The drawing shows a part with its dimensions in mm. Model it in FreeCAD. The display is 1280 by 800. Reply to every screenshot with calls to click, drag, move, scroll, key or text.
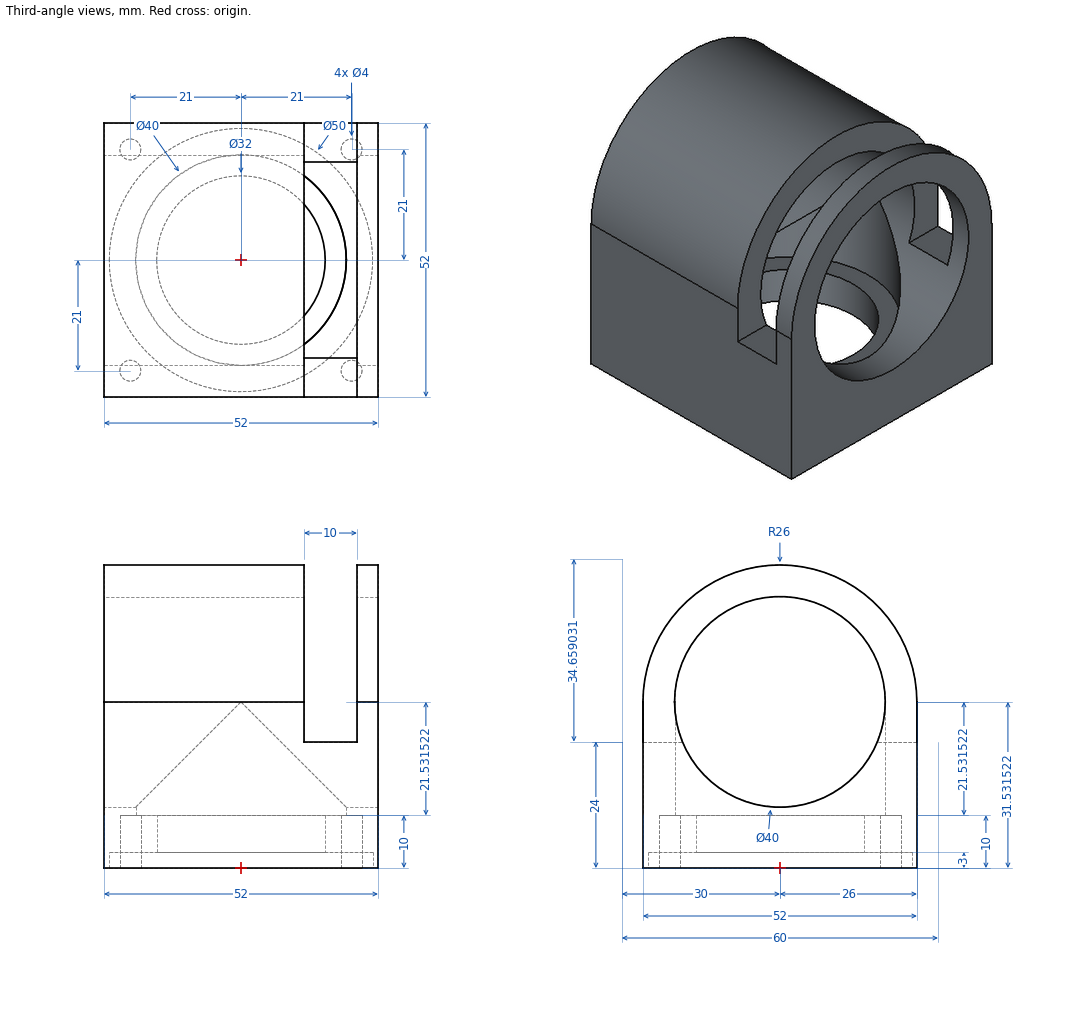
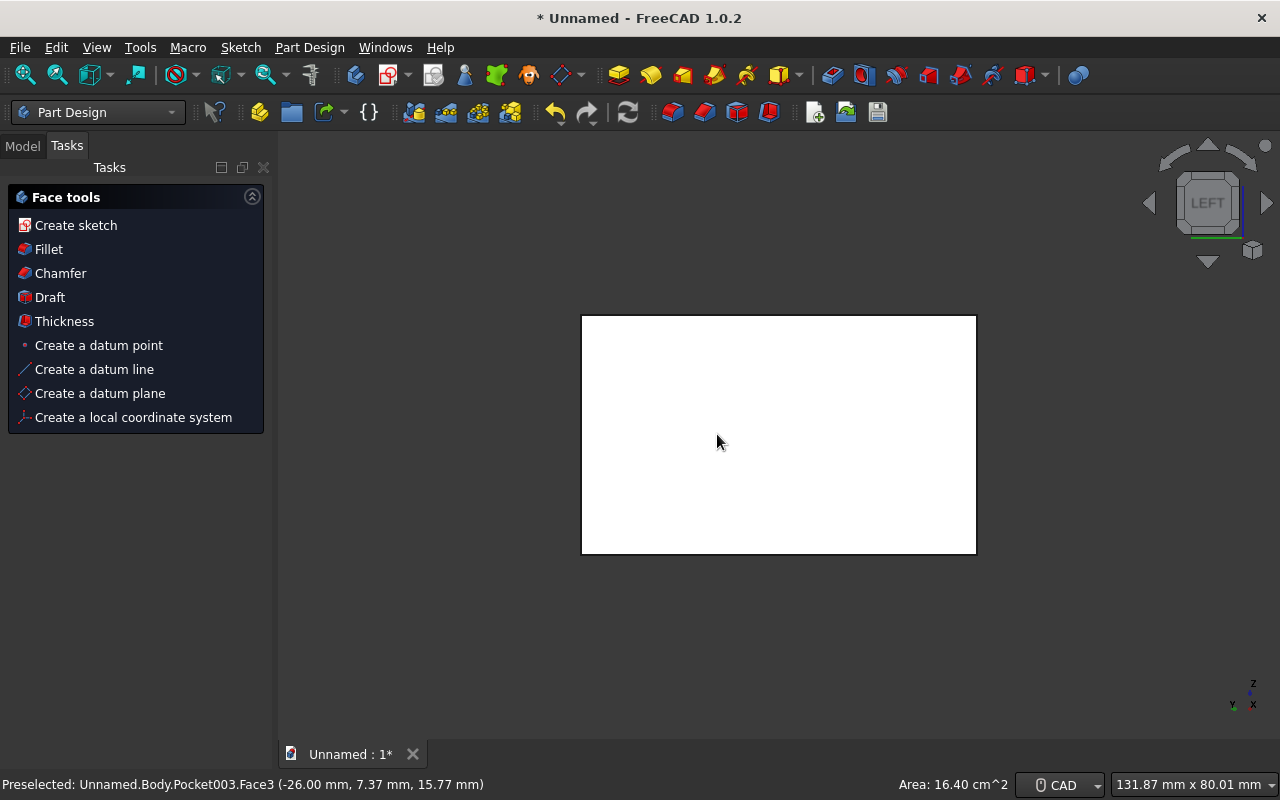
click(388, 76)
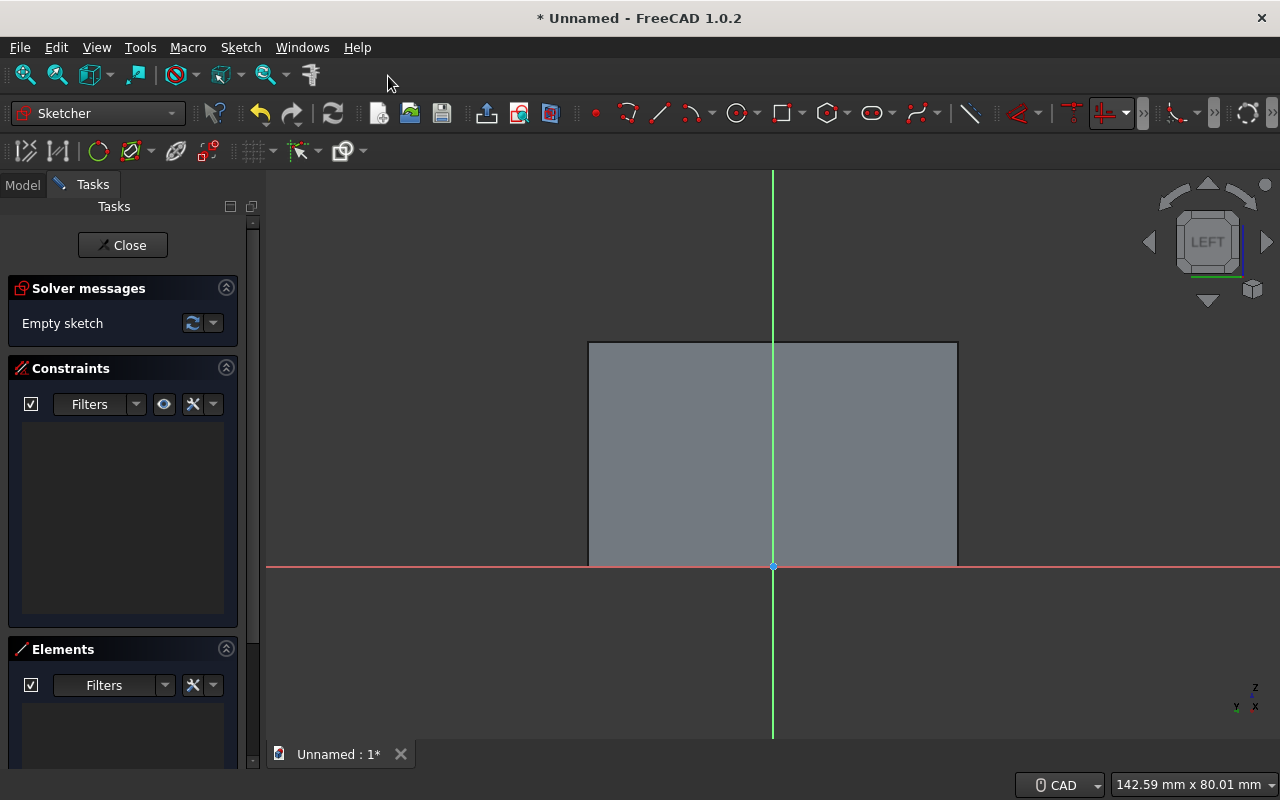
scroll(395, 711, down, 1)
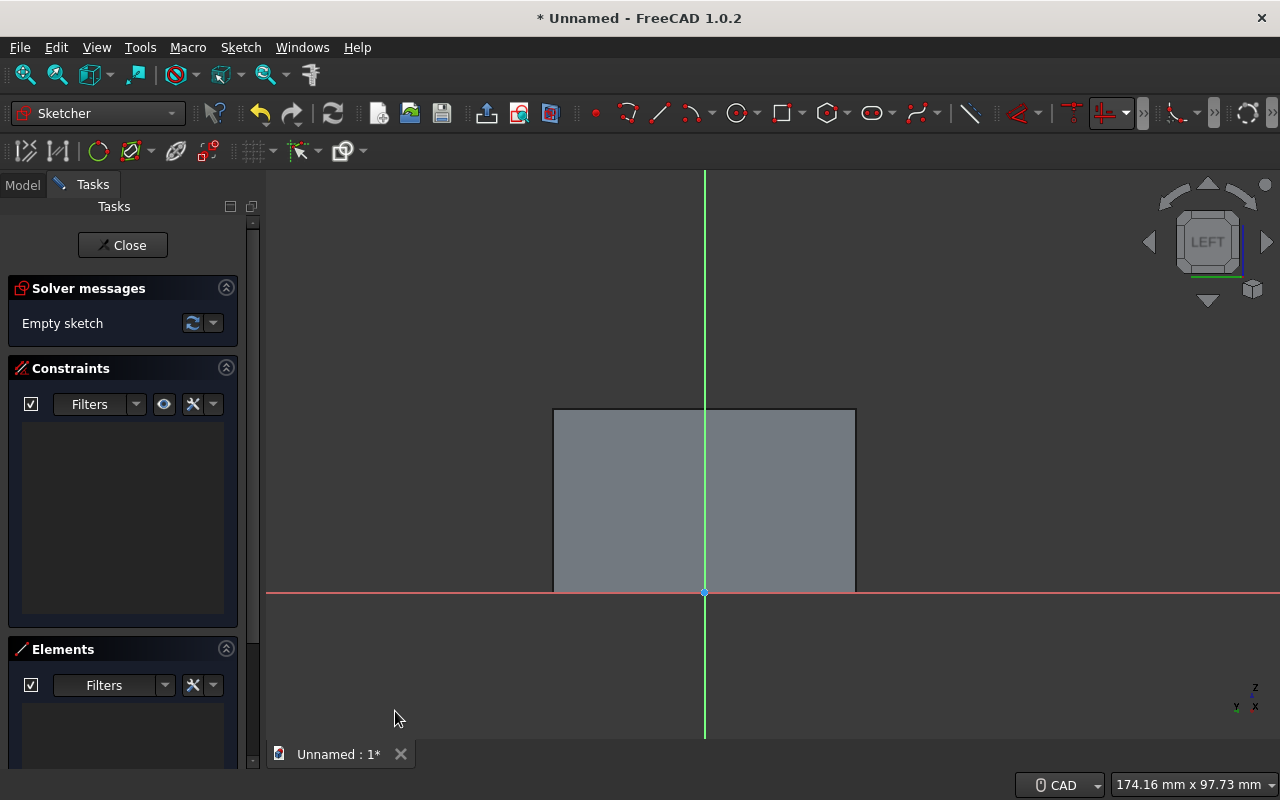
click(660, 114)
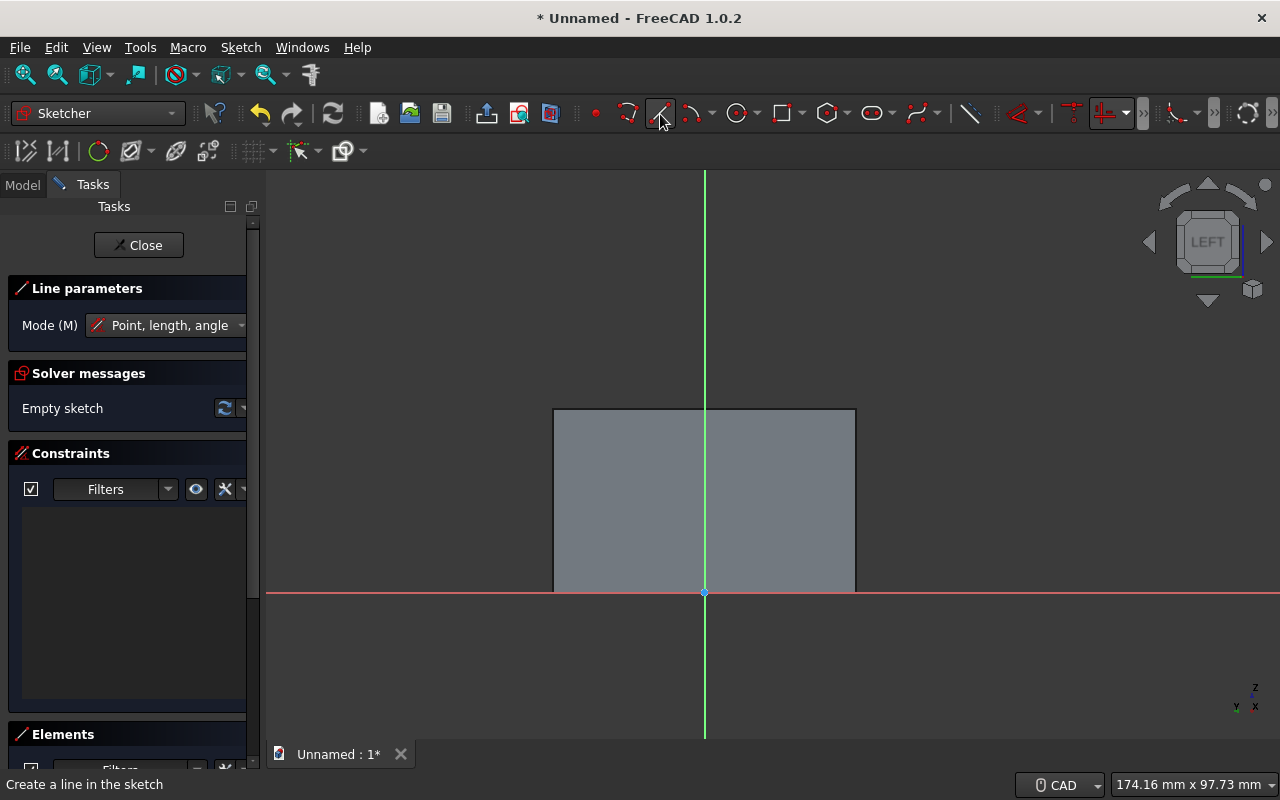
click(553, 409)
click(856, 409)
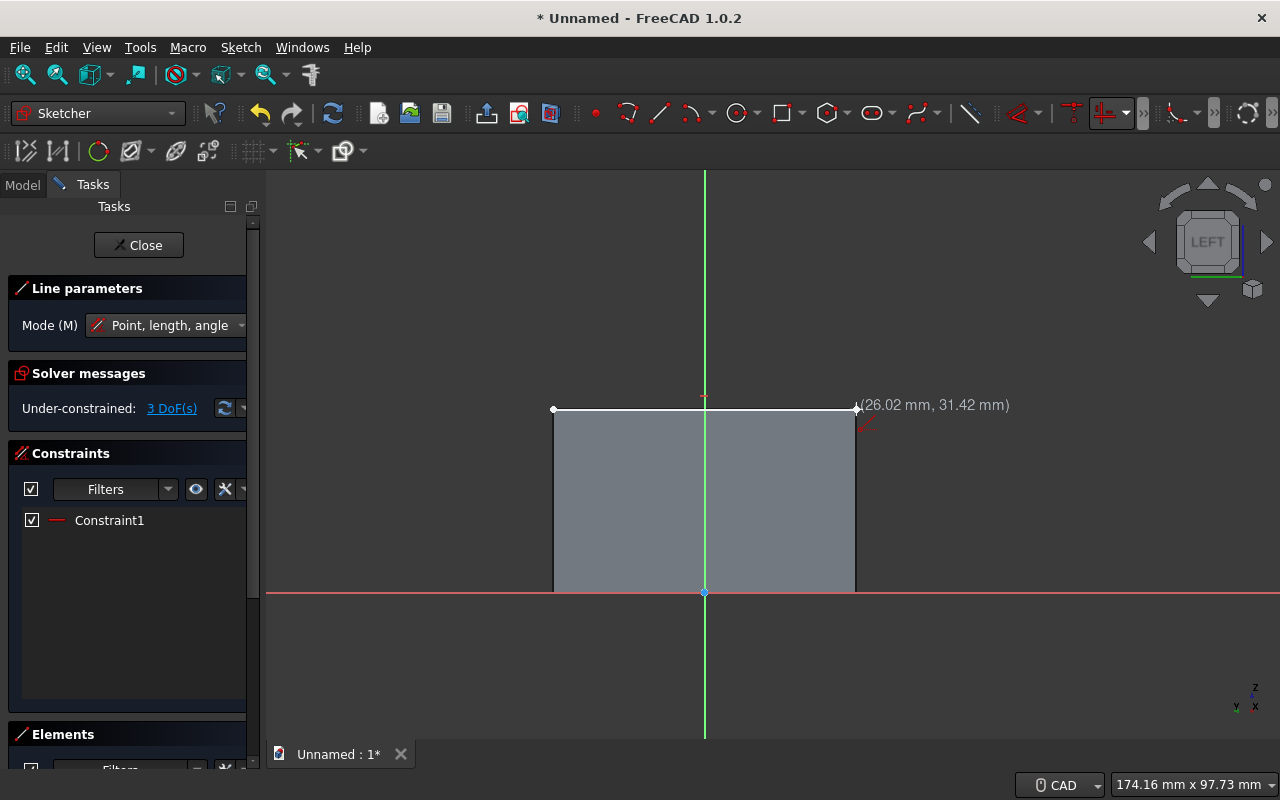
click(714, 114)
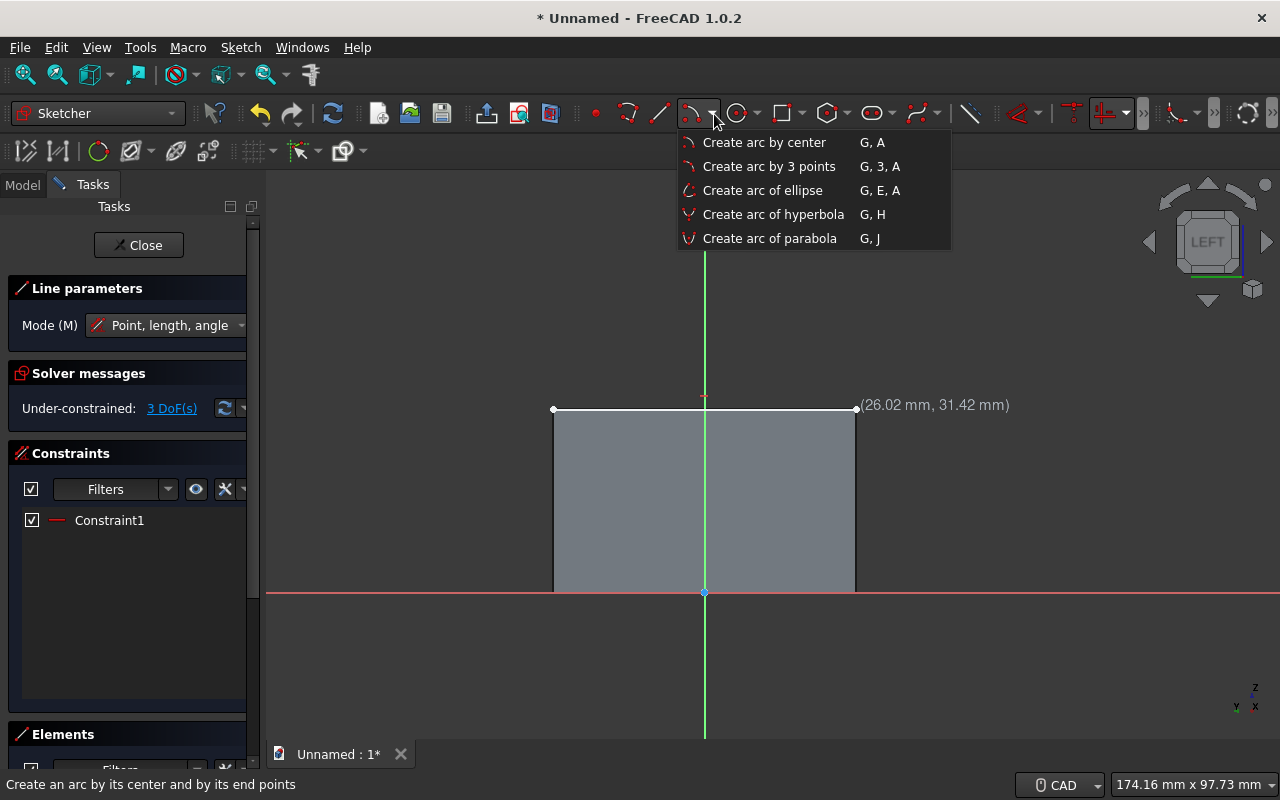
click(814, 166)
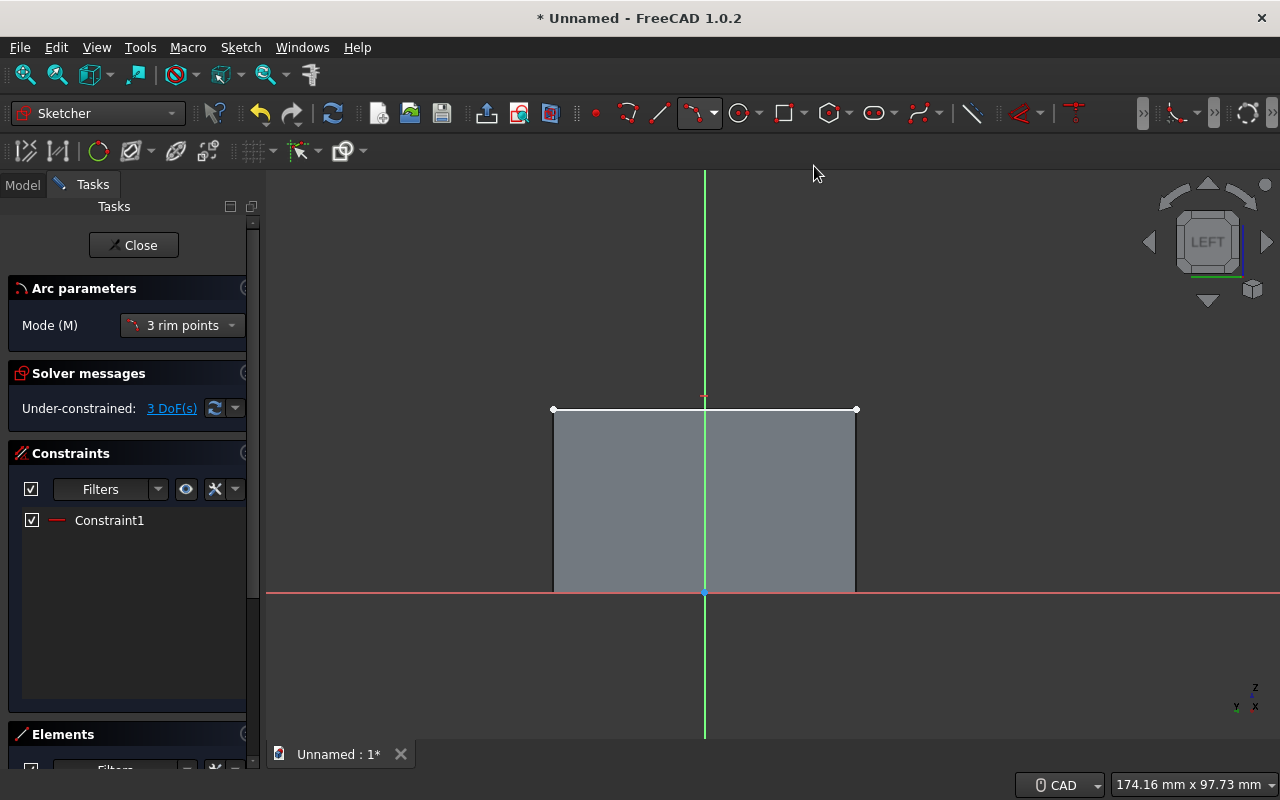
click(856, 410)
click(553, 410)
click(751, 265)
key(Escape)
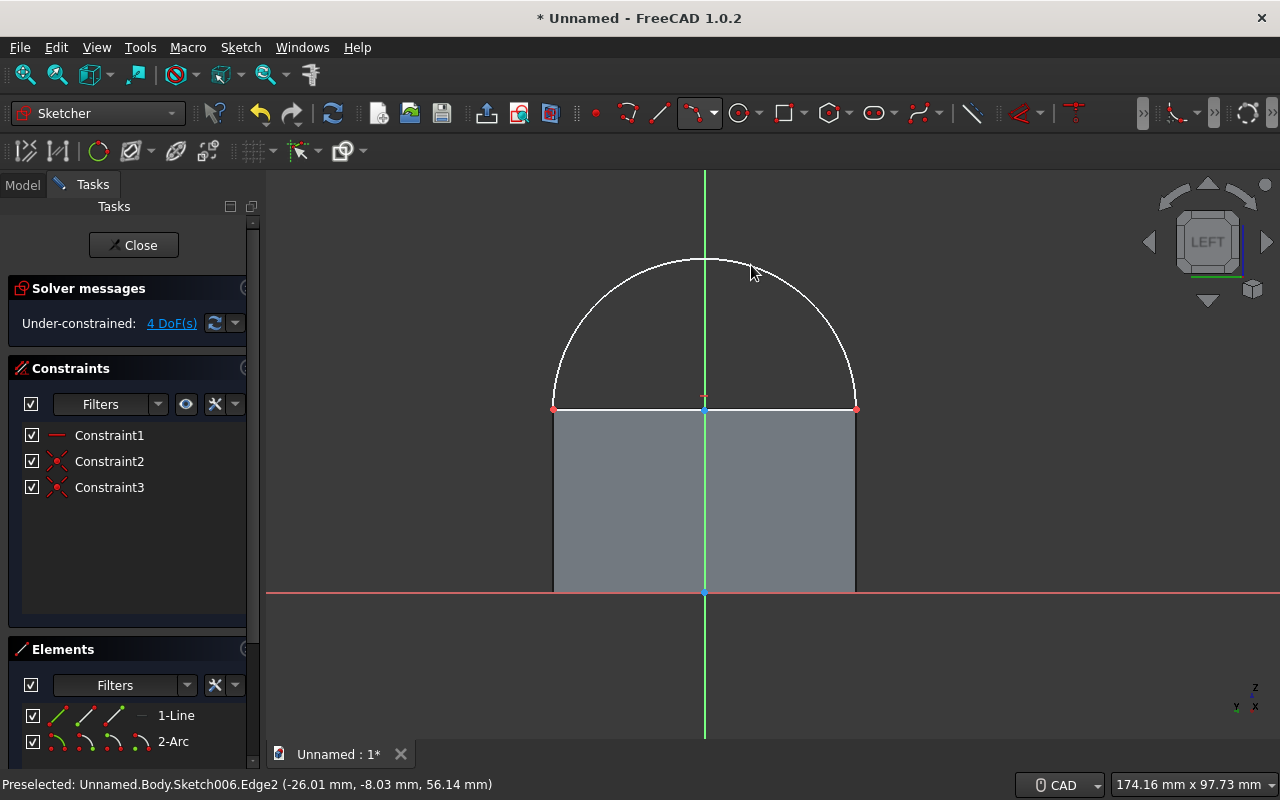
click(705, 410)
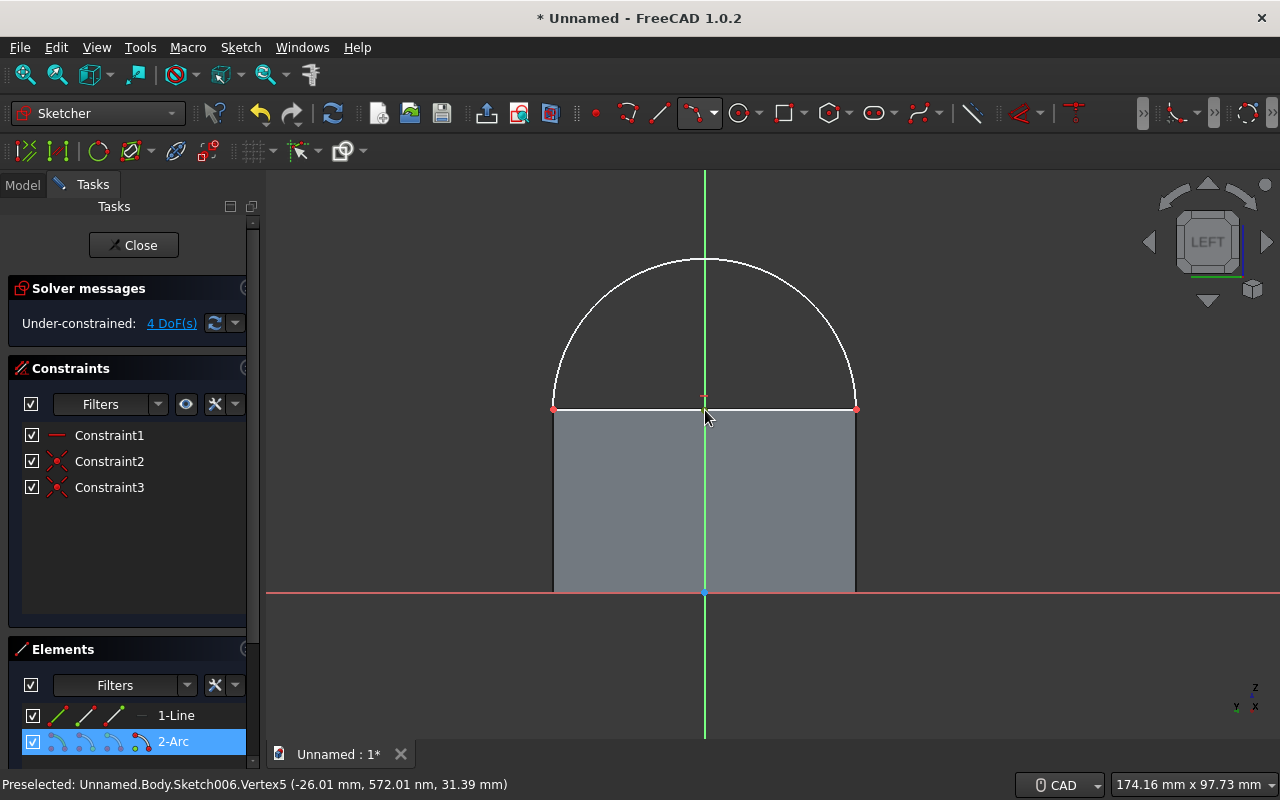
click(705, 674)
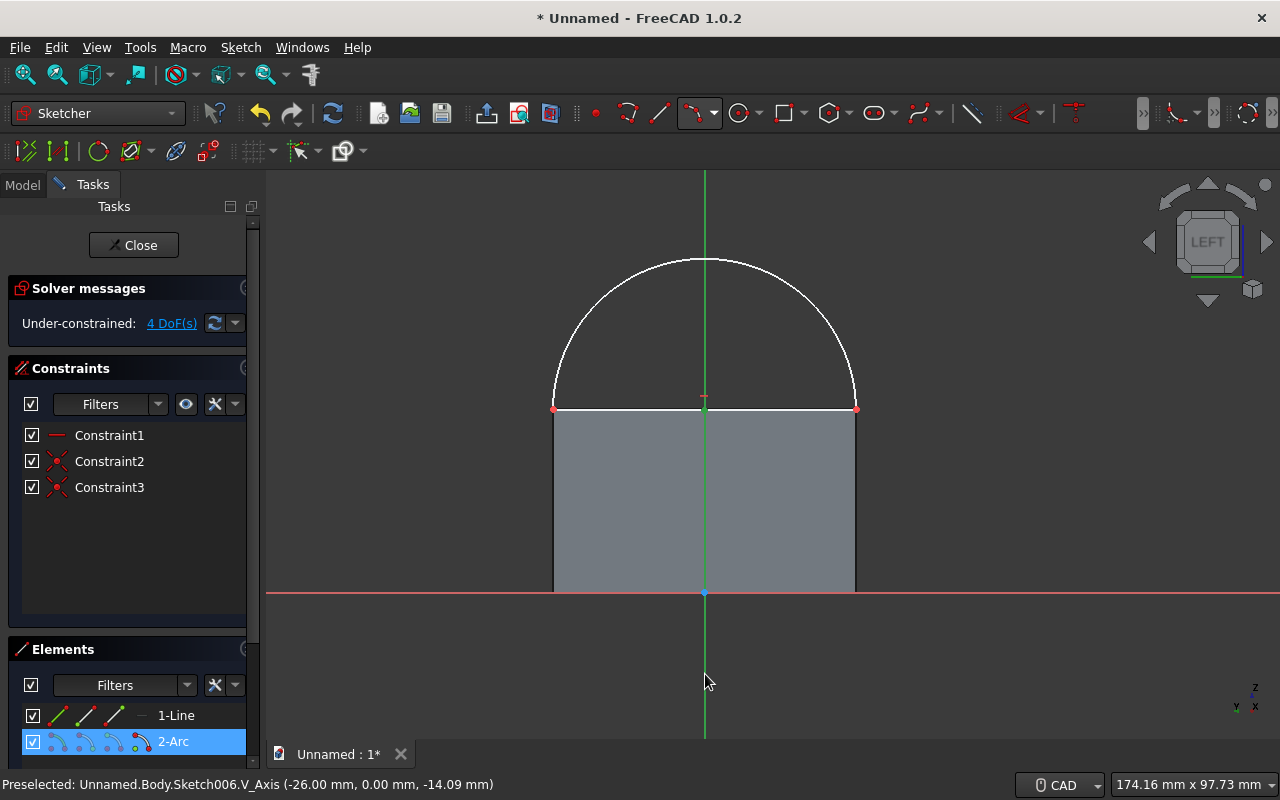
click(1074, 114)